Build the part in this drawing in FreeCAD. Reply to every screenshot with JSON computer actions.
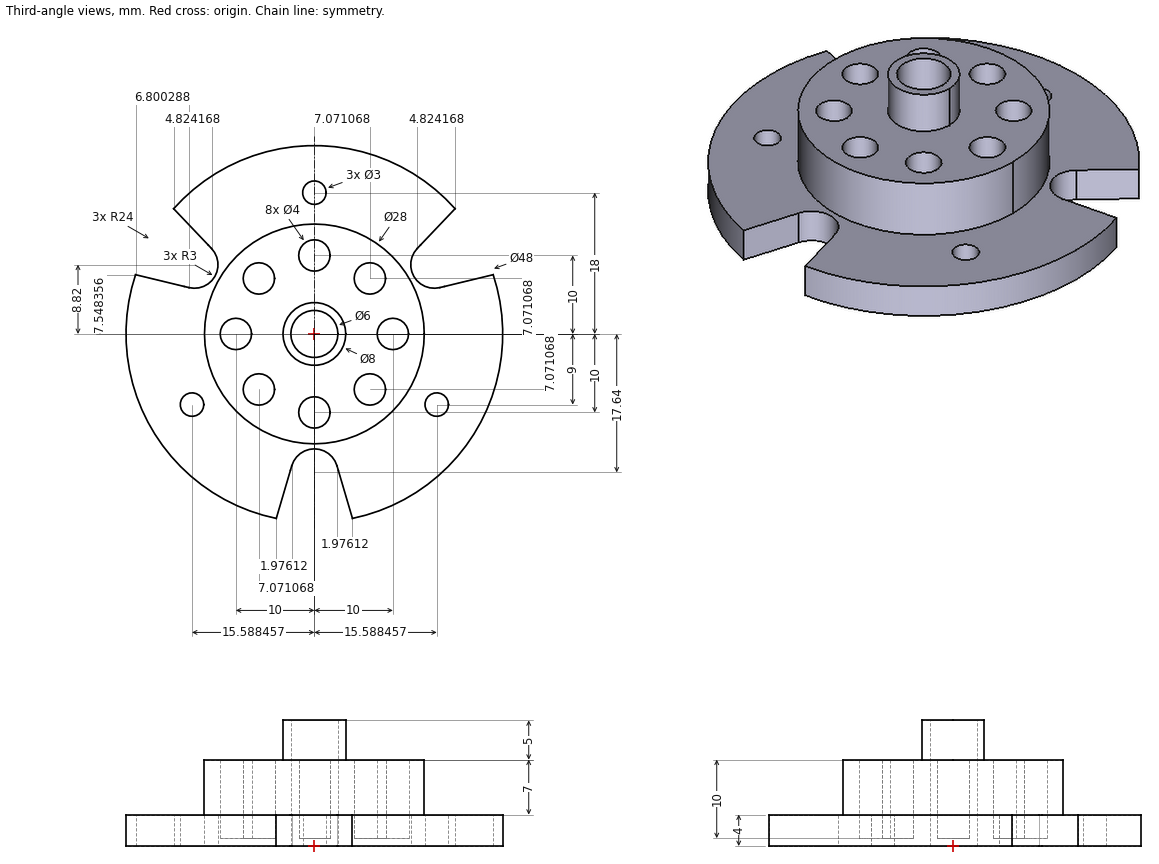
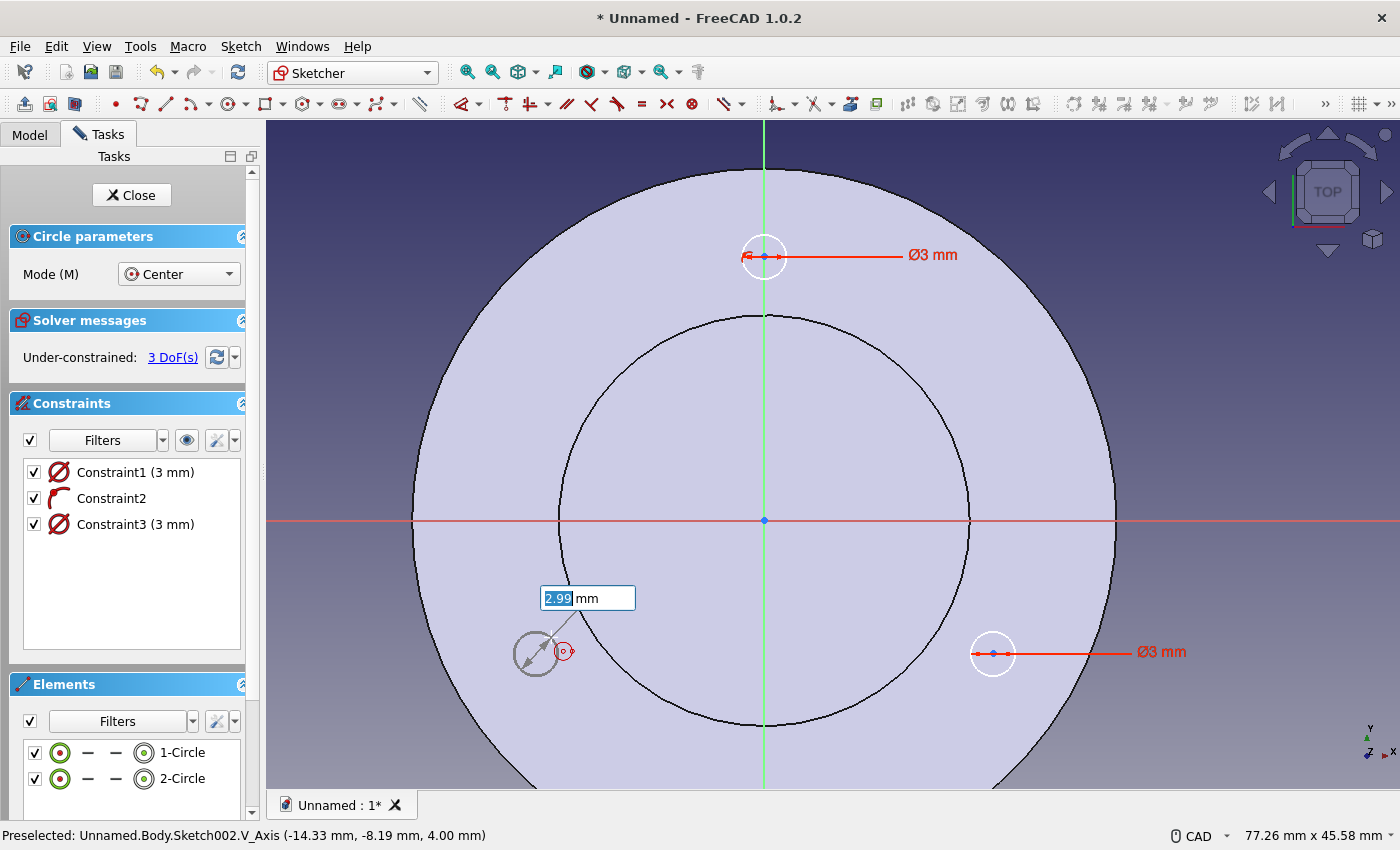
{"action": "type", "text": "3"}
{"action": "key", "text": "Return"}
{"action": "key", "text": "Escape"}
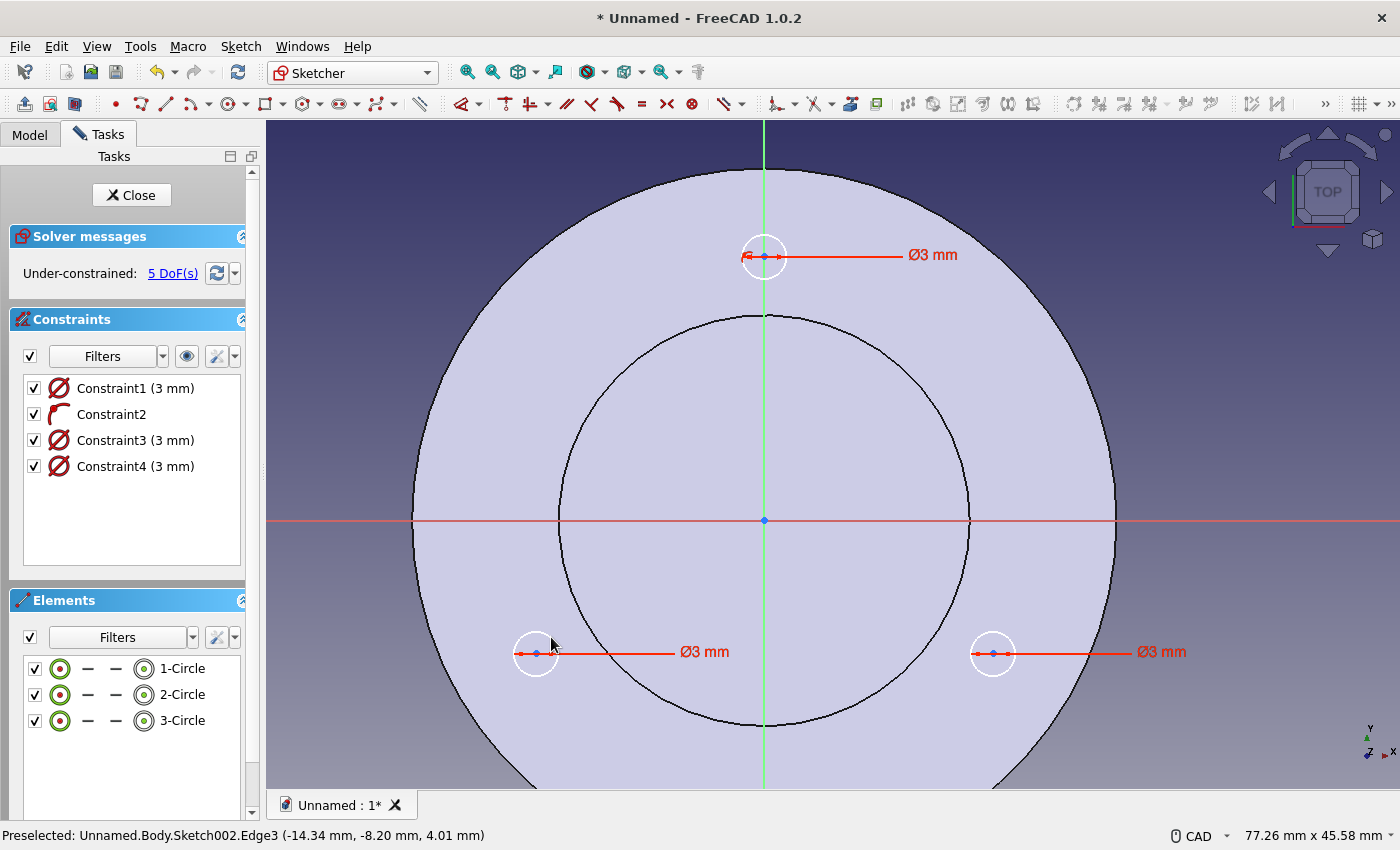
{"action": "left_click", "coordinate": [993, 654]}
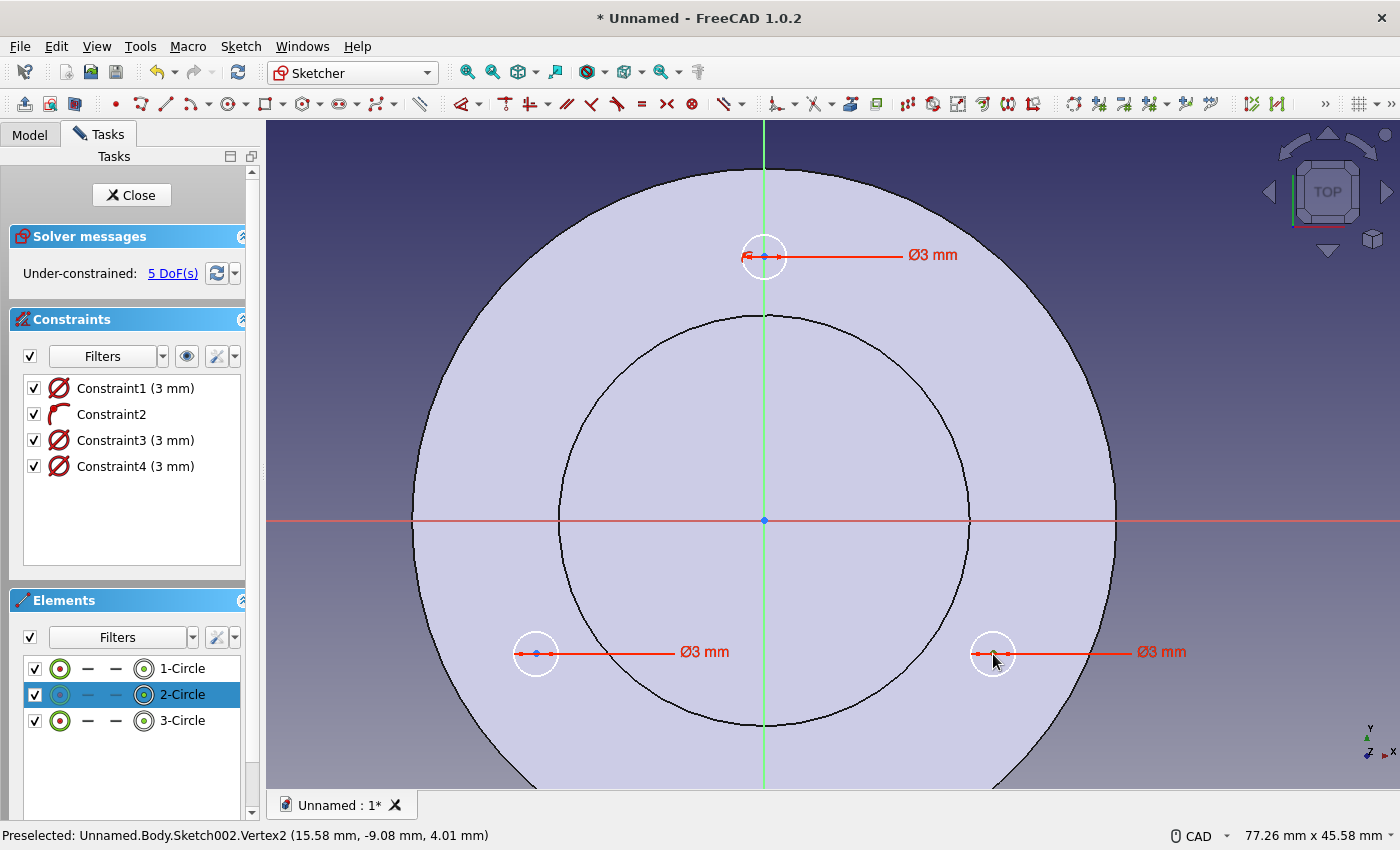
{"action": "left_click", "coordinate": [536, 654]}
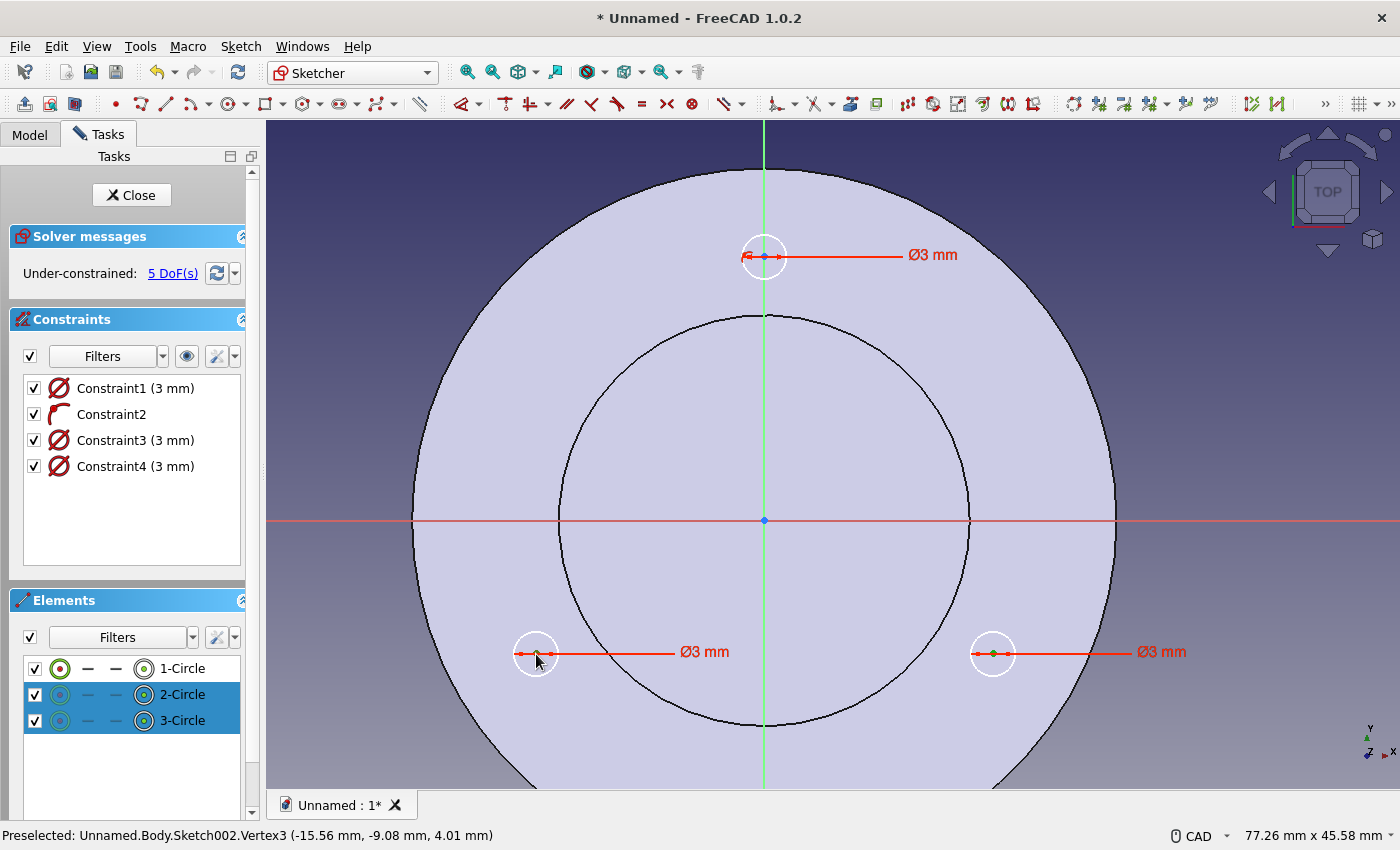
{"action": "left_click", "coordinate": [548, 104]}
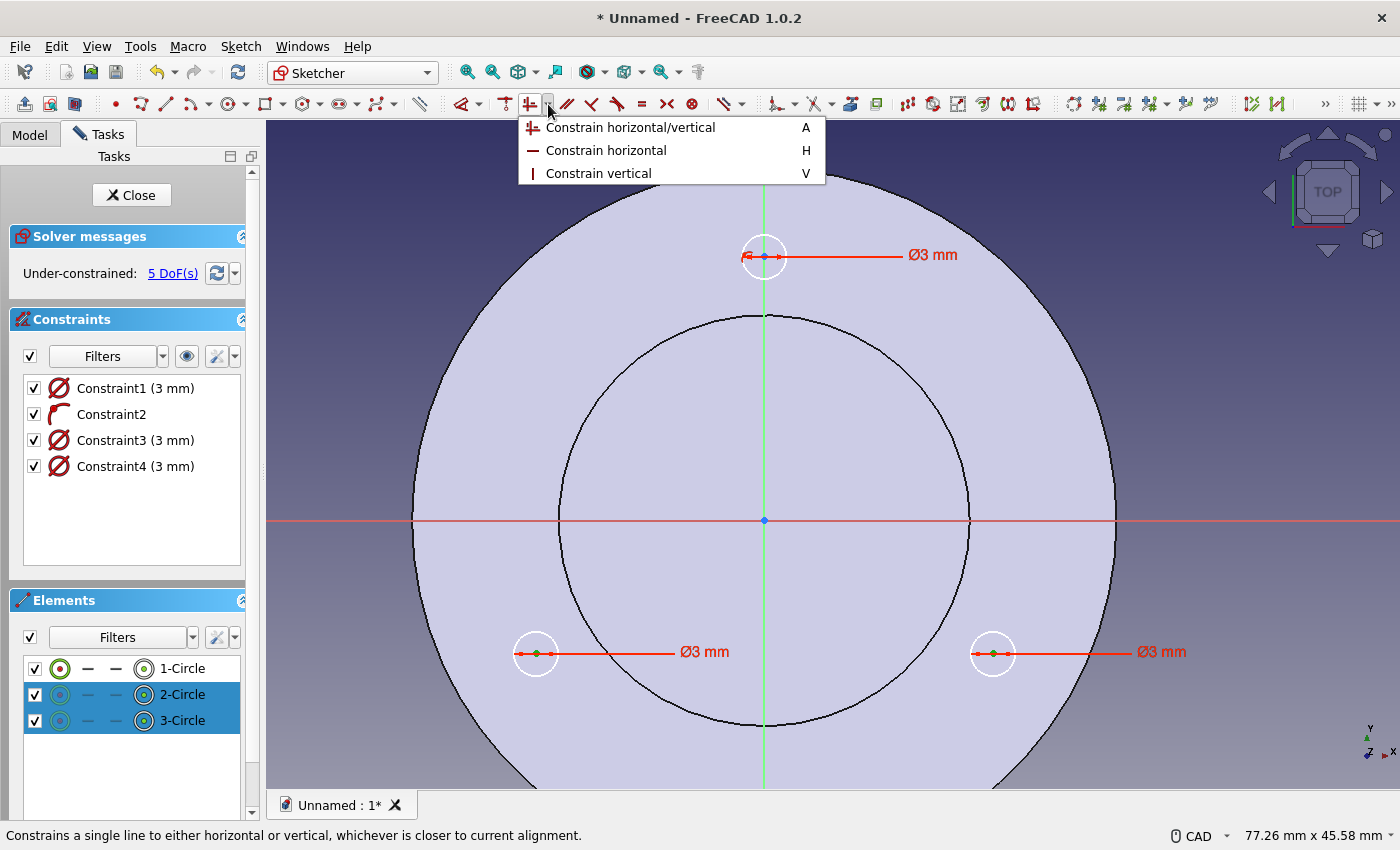
{"action": "left_click", "coordinate": [672, 150]}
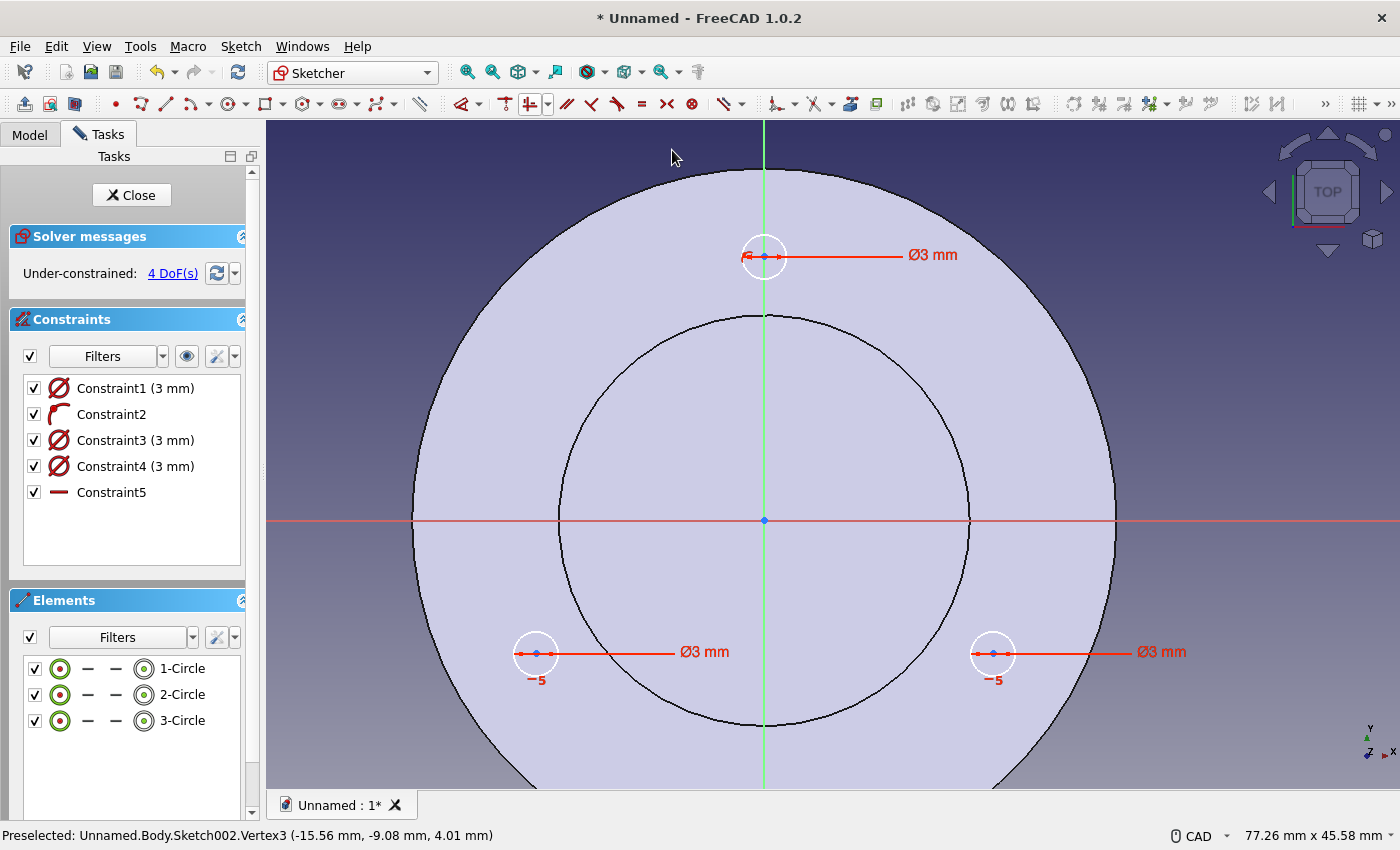
{"action": "left_click", "coordinate": [460, 104]}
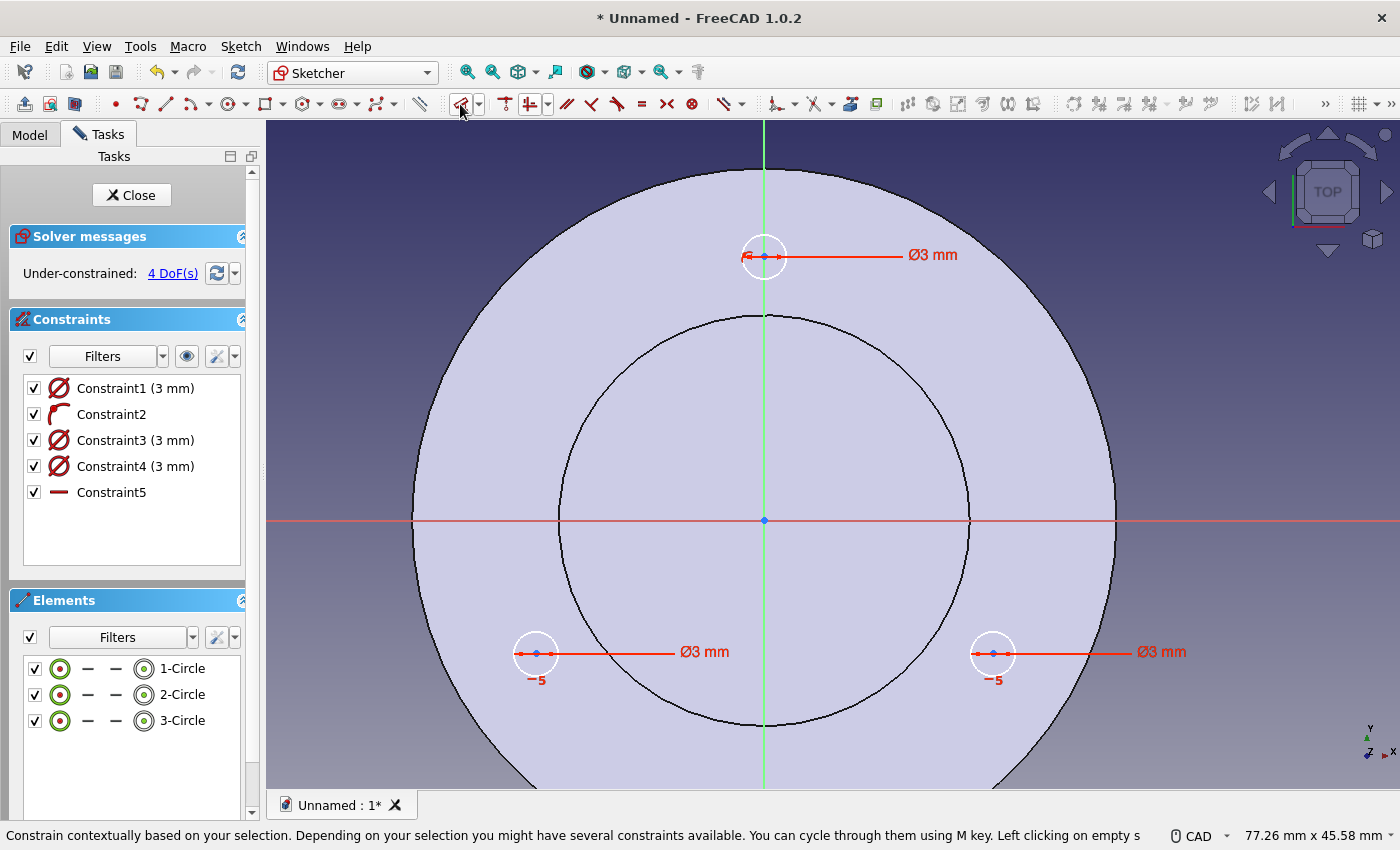
{"action": "left_click", "coordinate": [993, 654]}
{"action": "left_click", "coordinate": [1027, 587]}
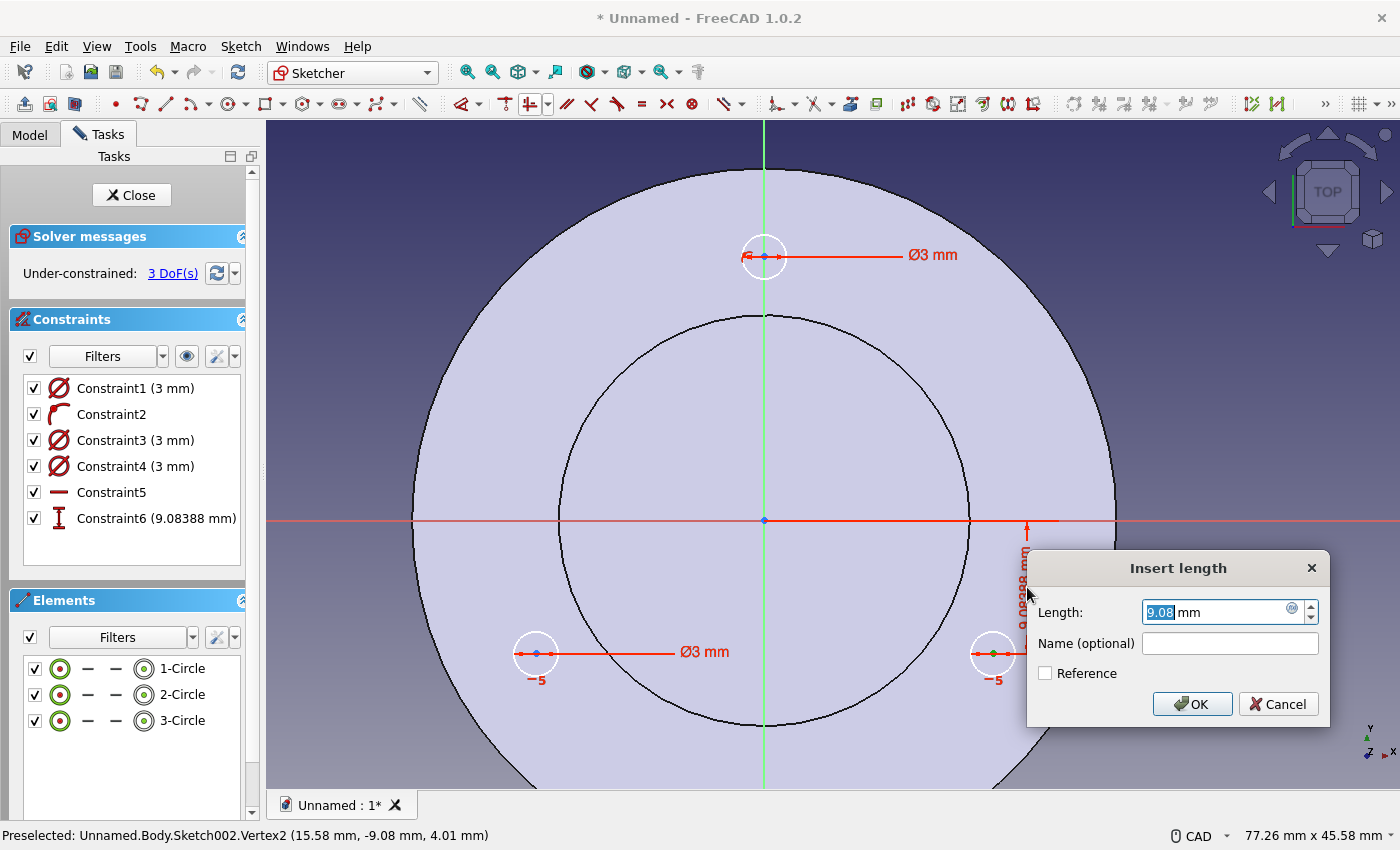
{"action": "type", "text": "9"}
{"action": "key", "text": "Return"}